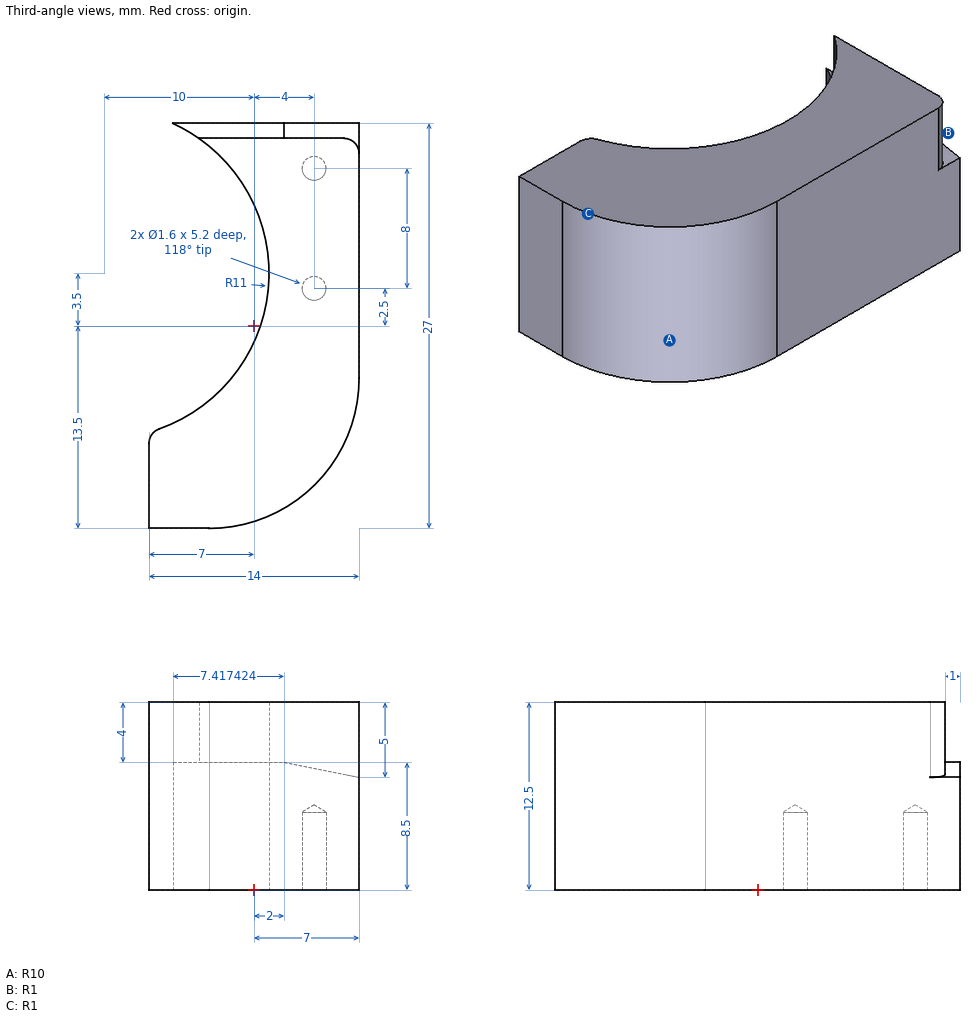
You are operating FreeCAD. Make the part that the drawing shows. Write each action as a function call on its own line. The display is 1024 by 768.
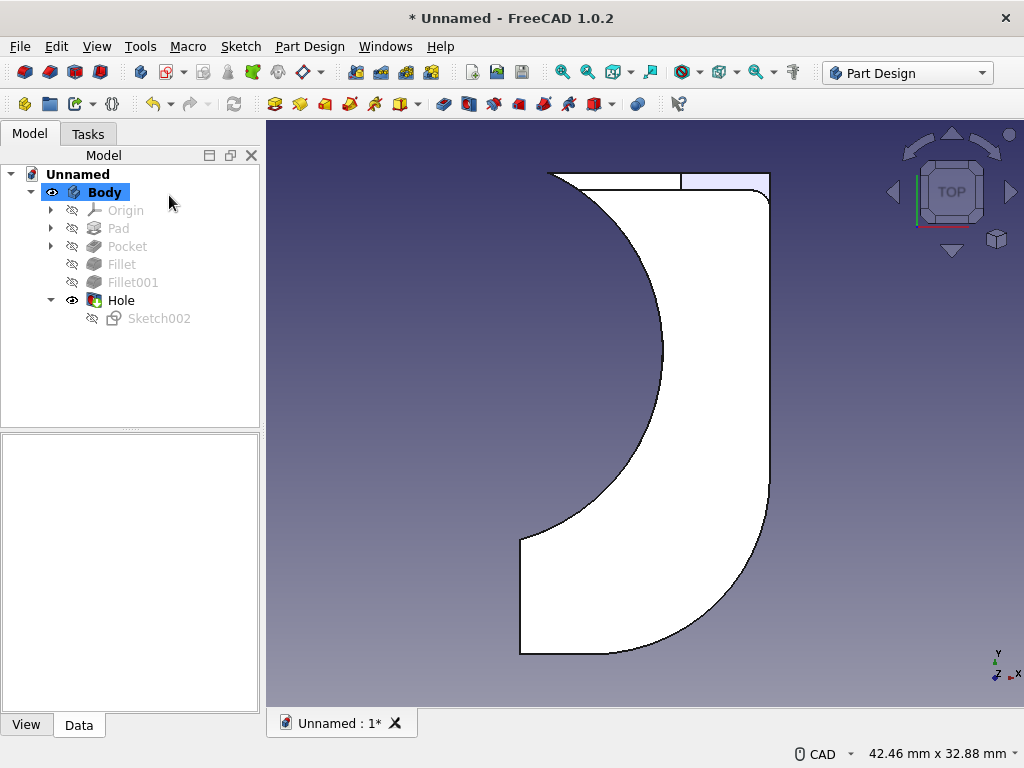
key(1)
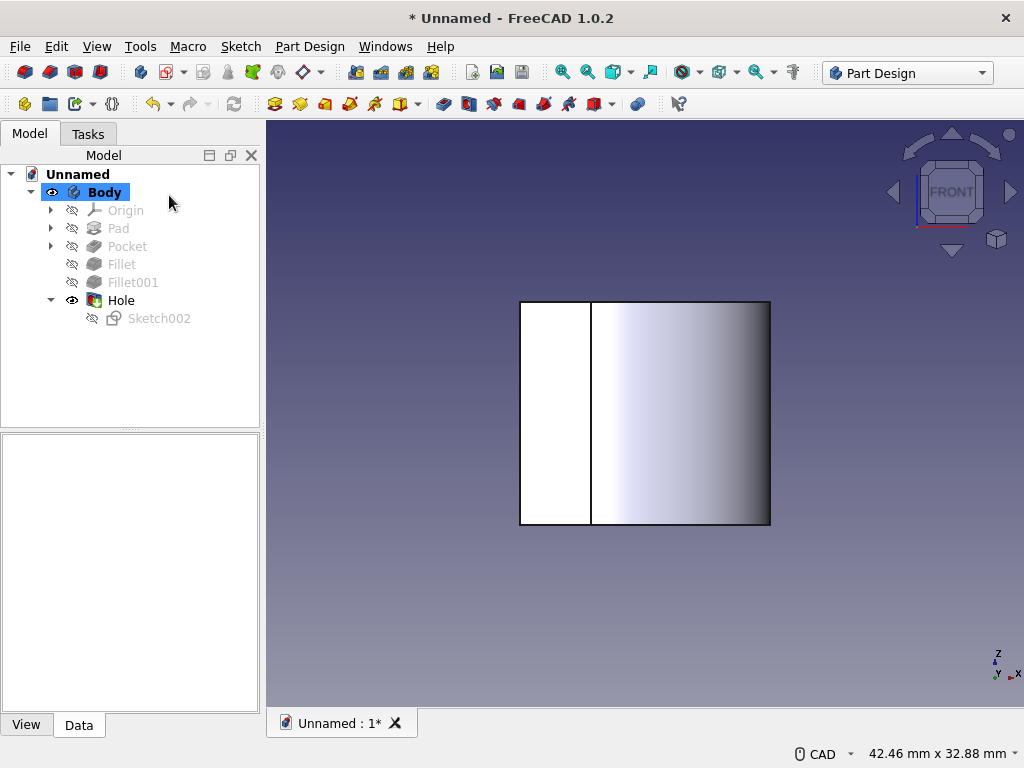
click(563, 72)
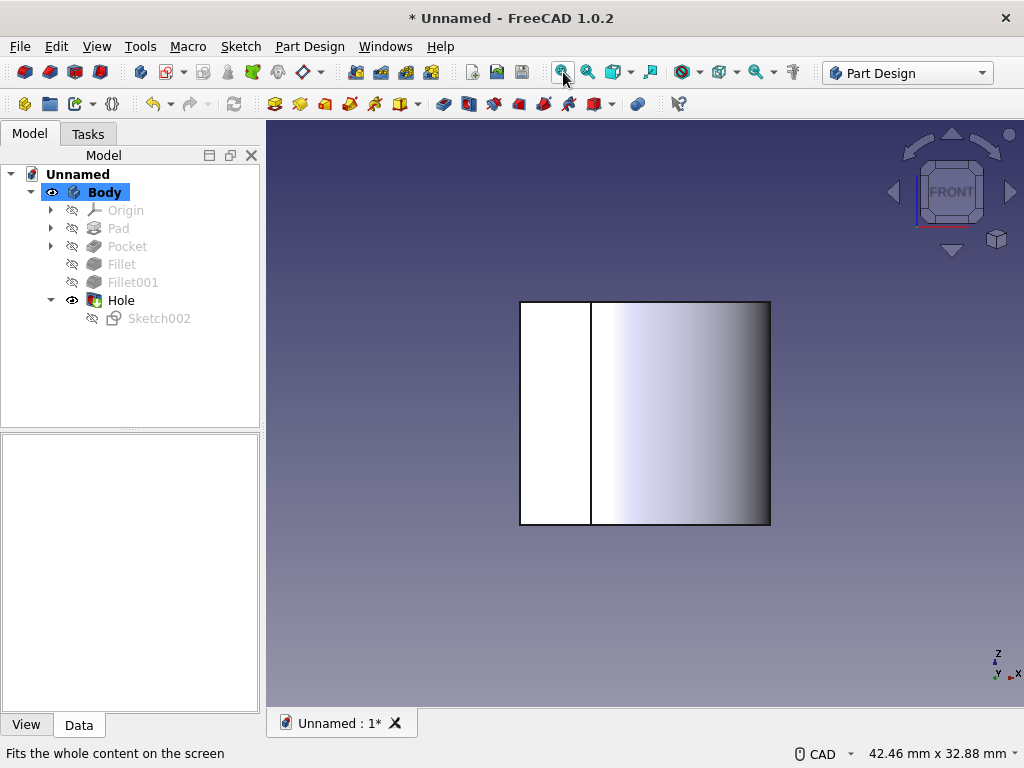
key(3)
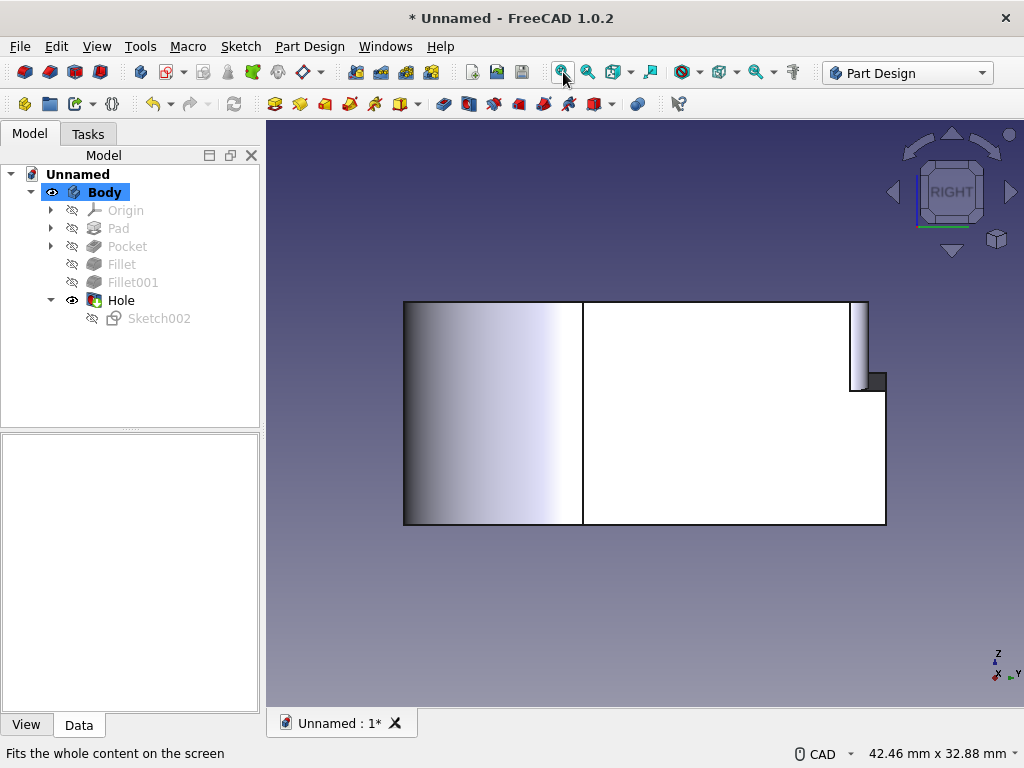
key(5)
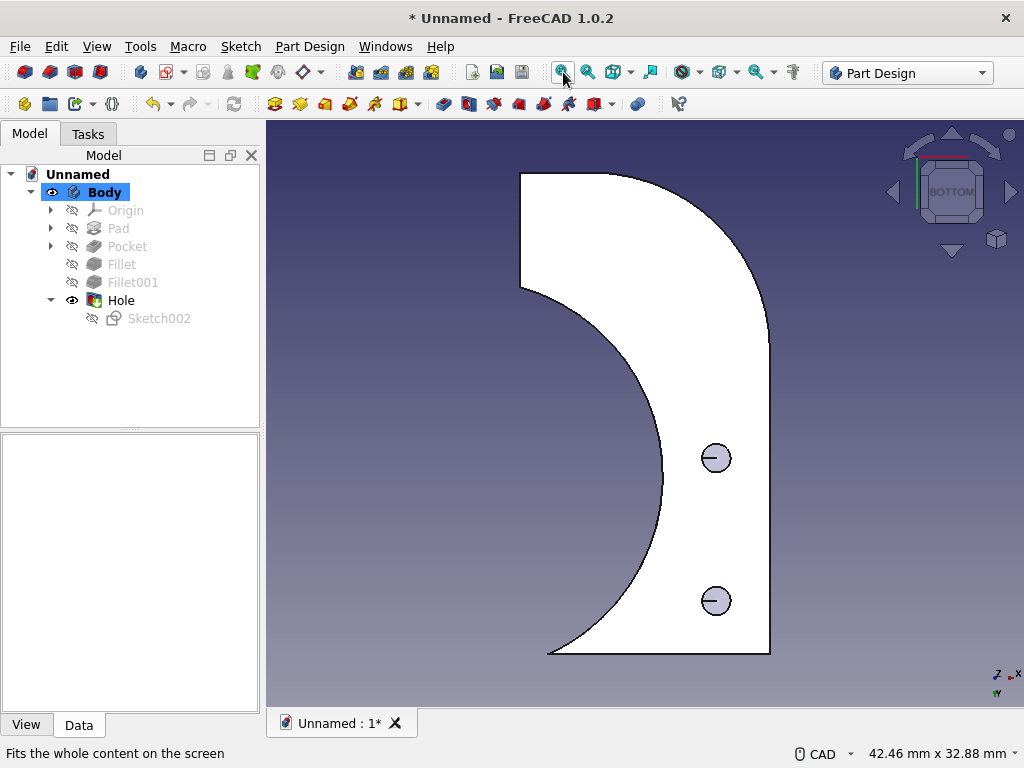
key(4)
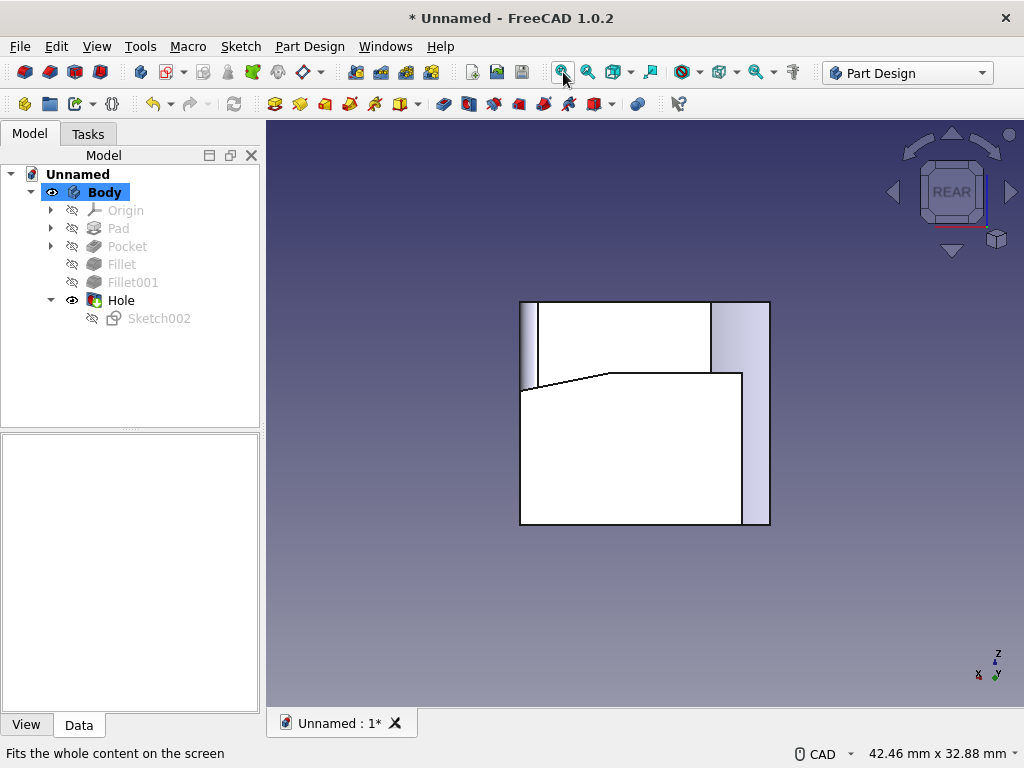
click(563, 72)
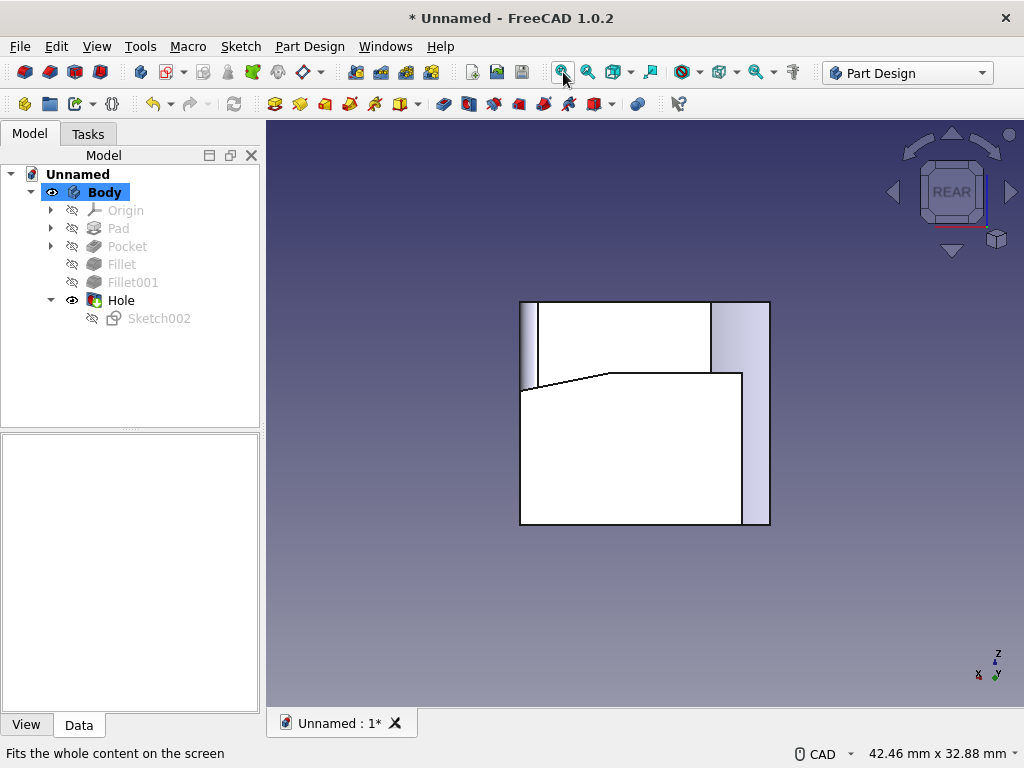
key(6)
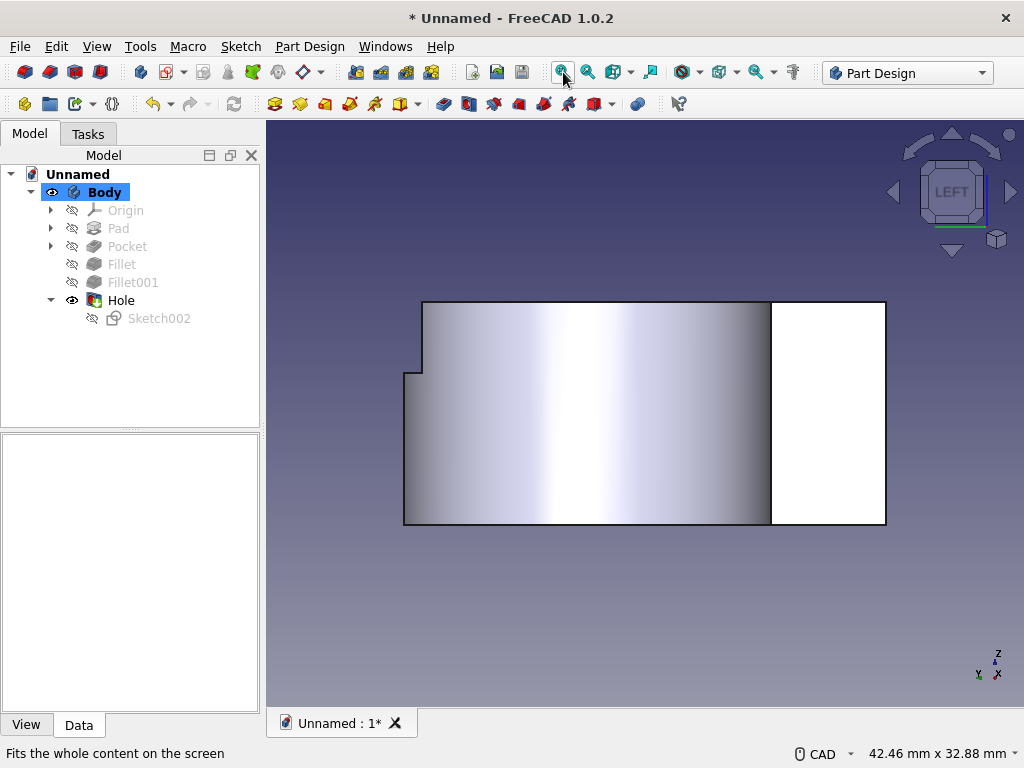
click(771, 412)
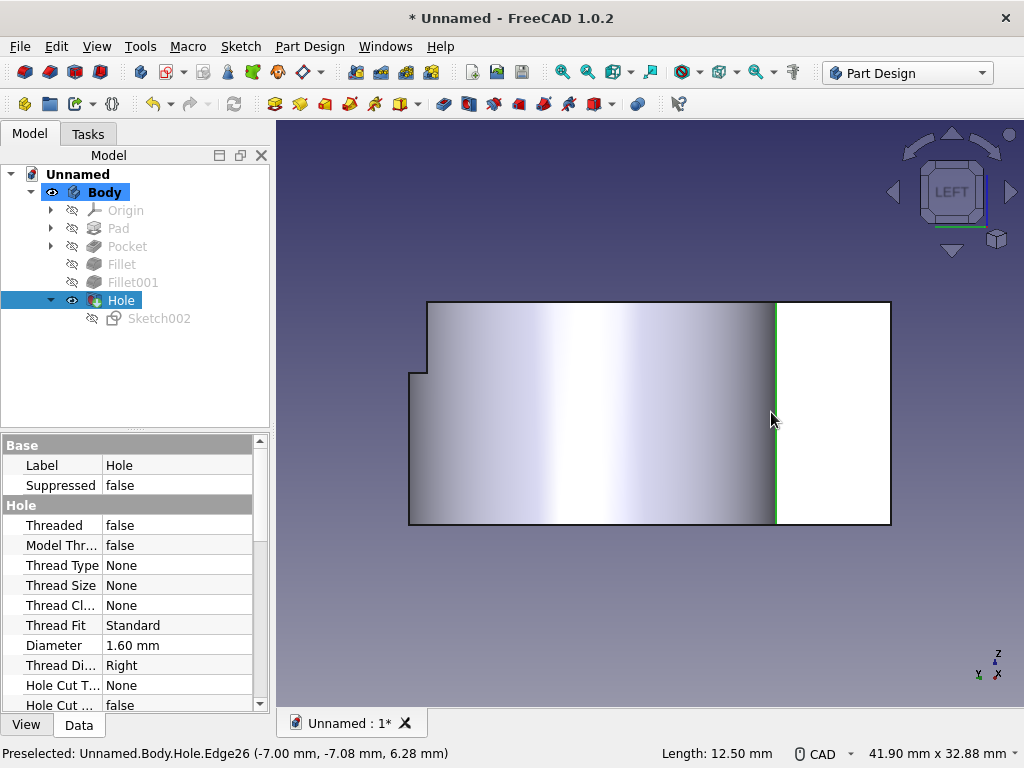
click(25, 72)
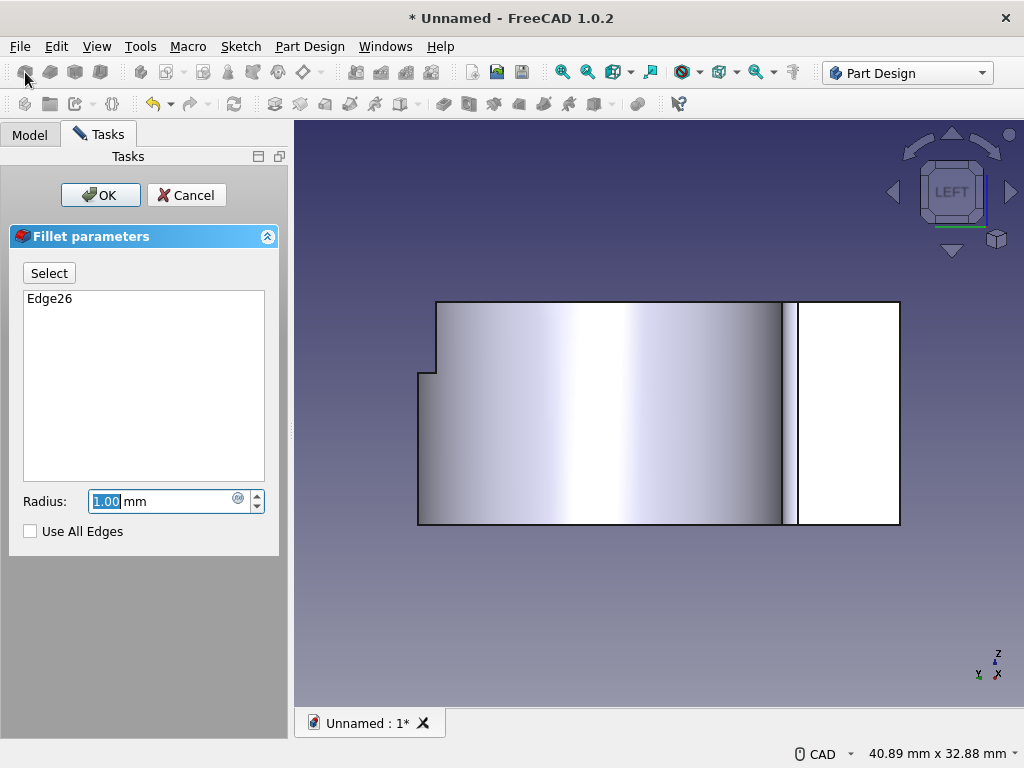
text(1)
key(Tab)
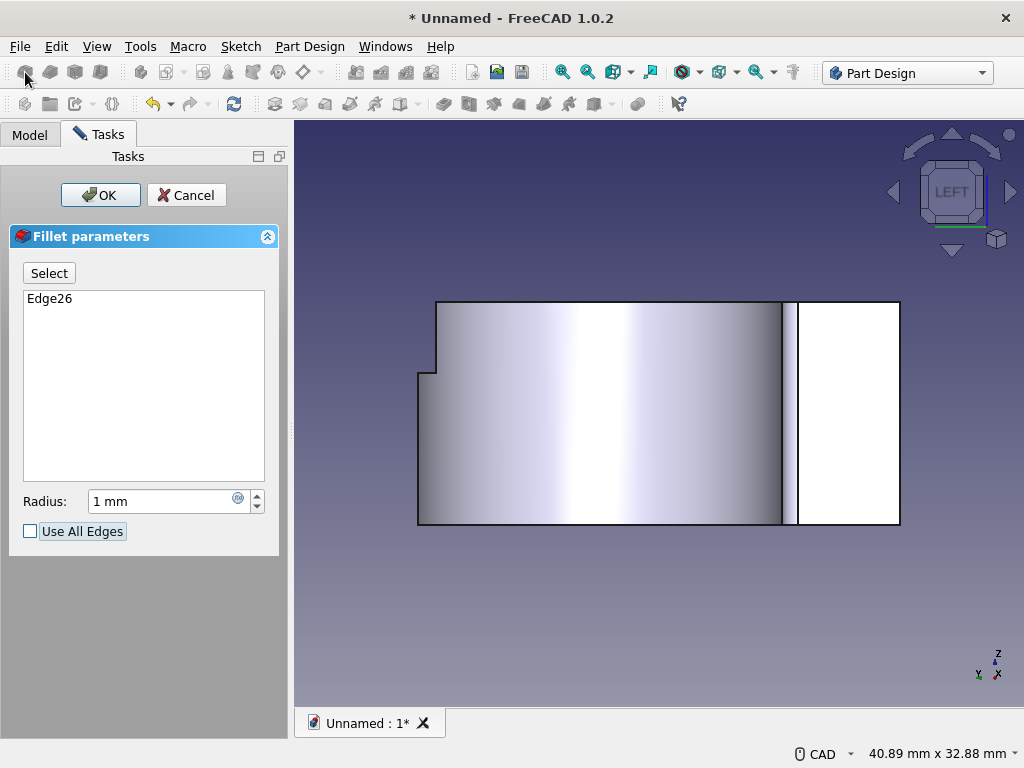
click(101, 195)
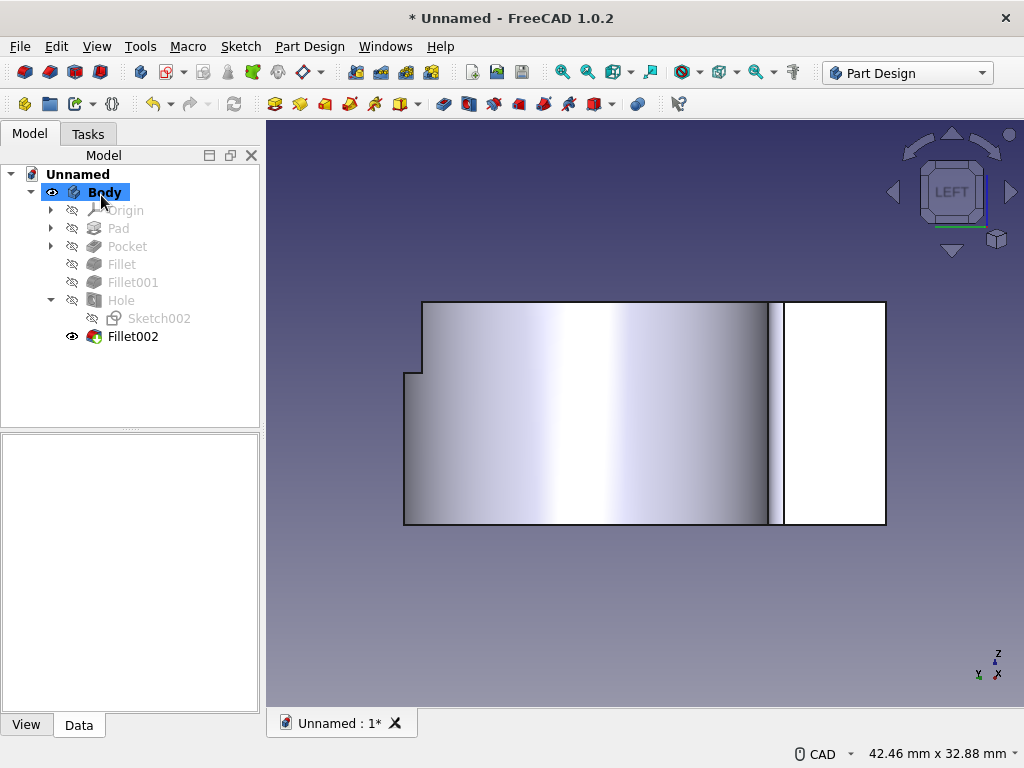
key(0)